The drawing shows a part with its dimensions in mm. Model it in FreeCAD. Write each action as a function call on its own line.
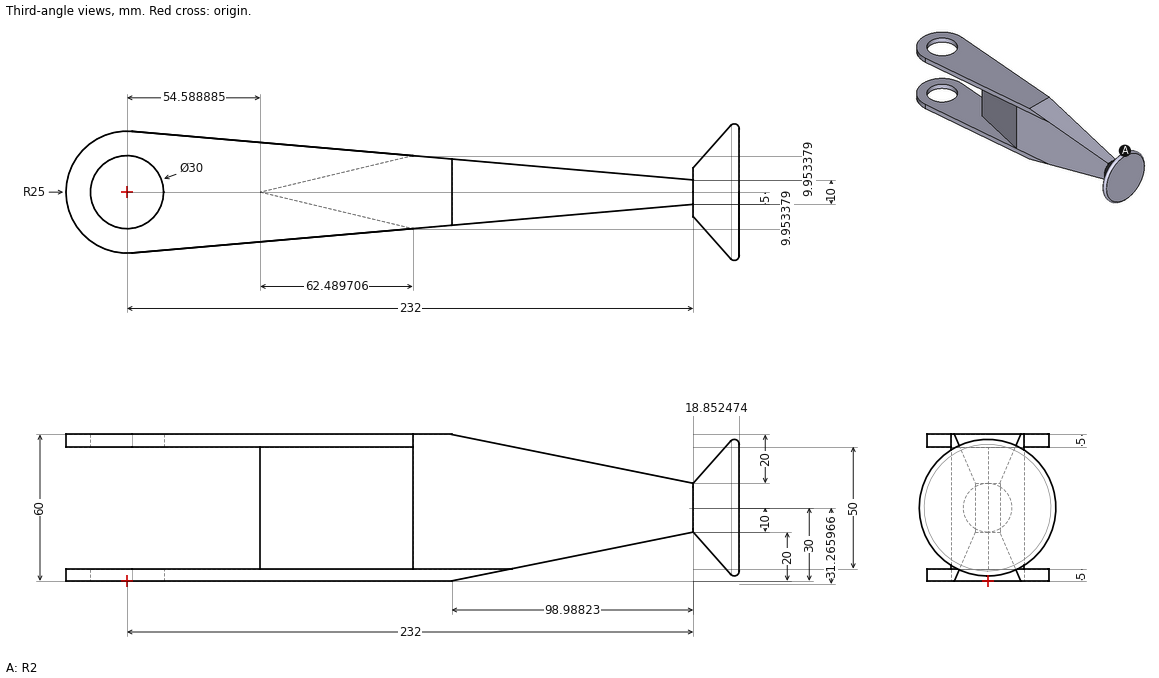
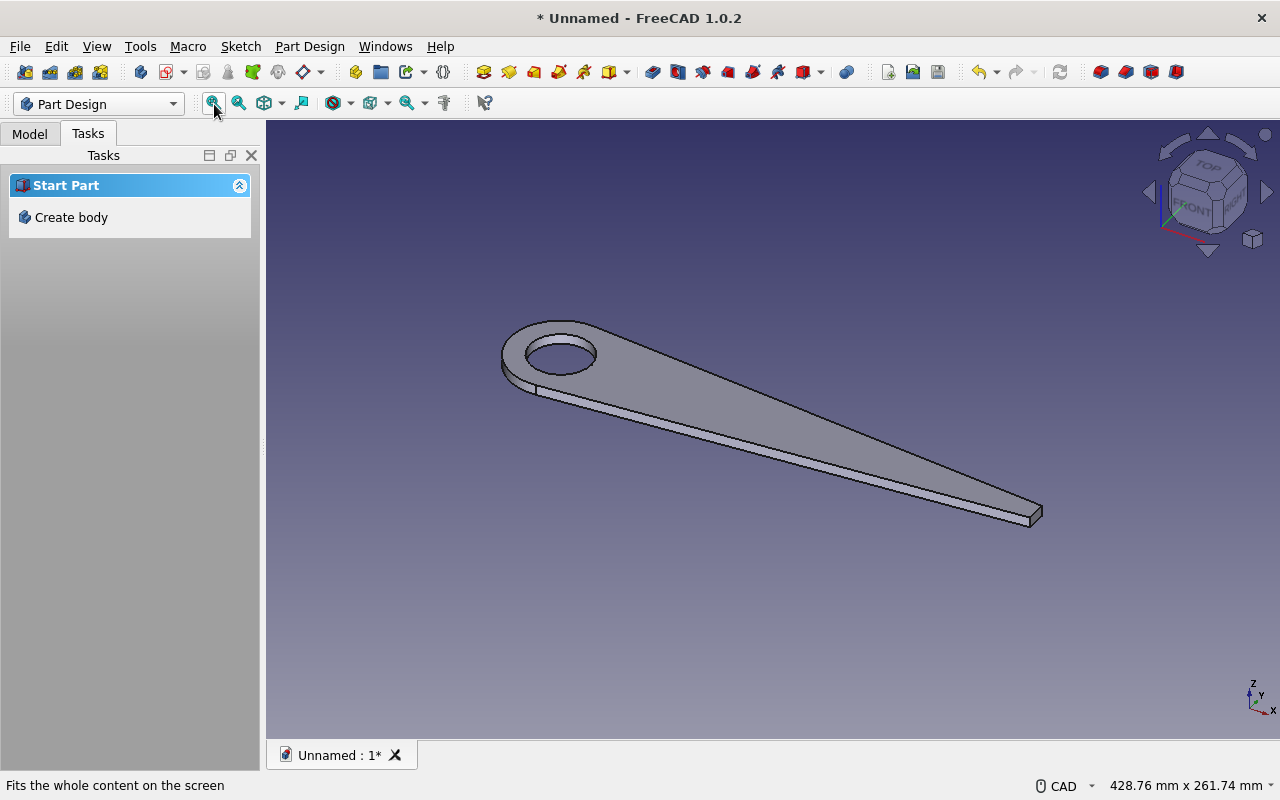
click(698, 399)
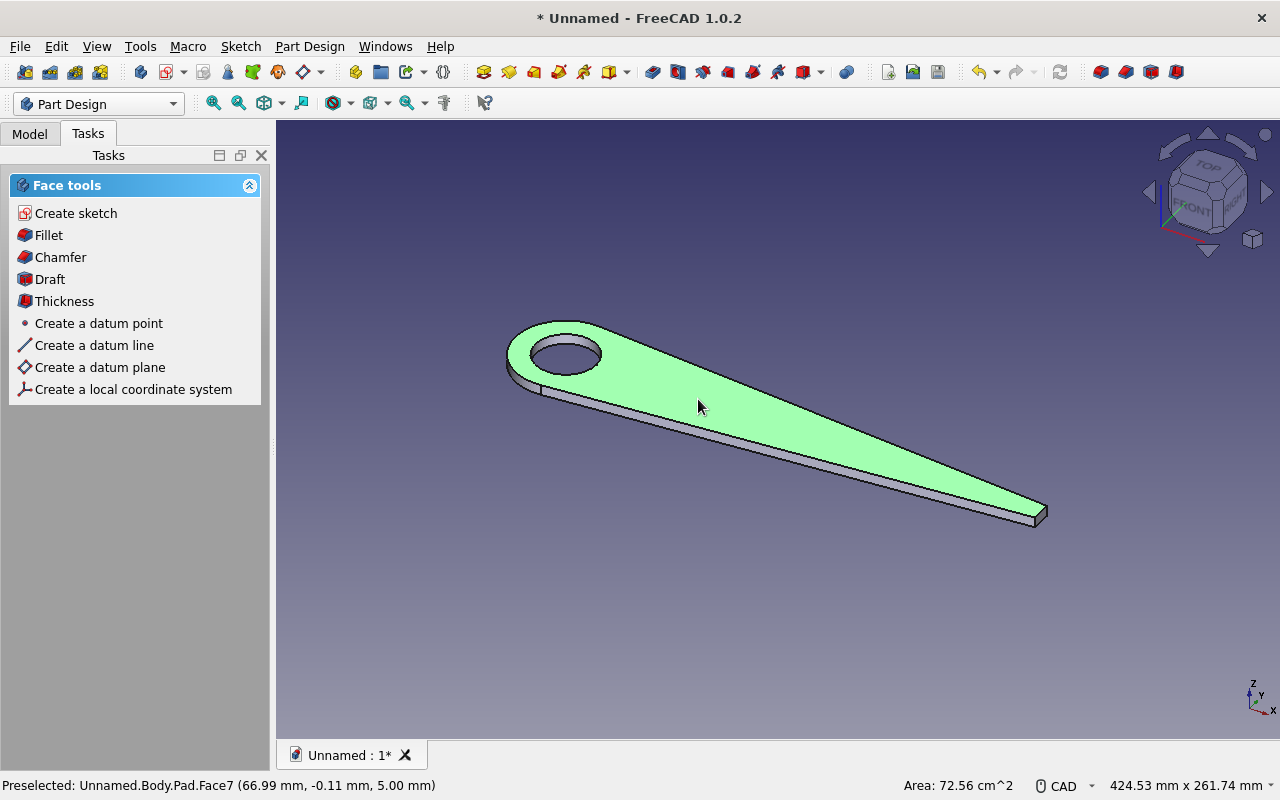
click(166, 72)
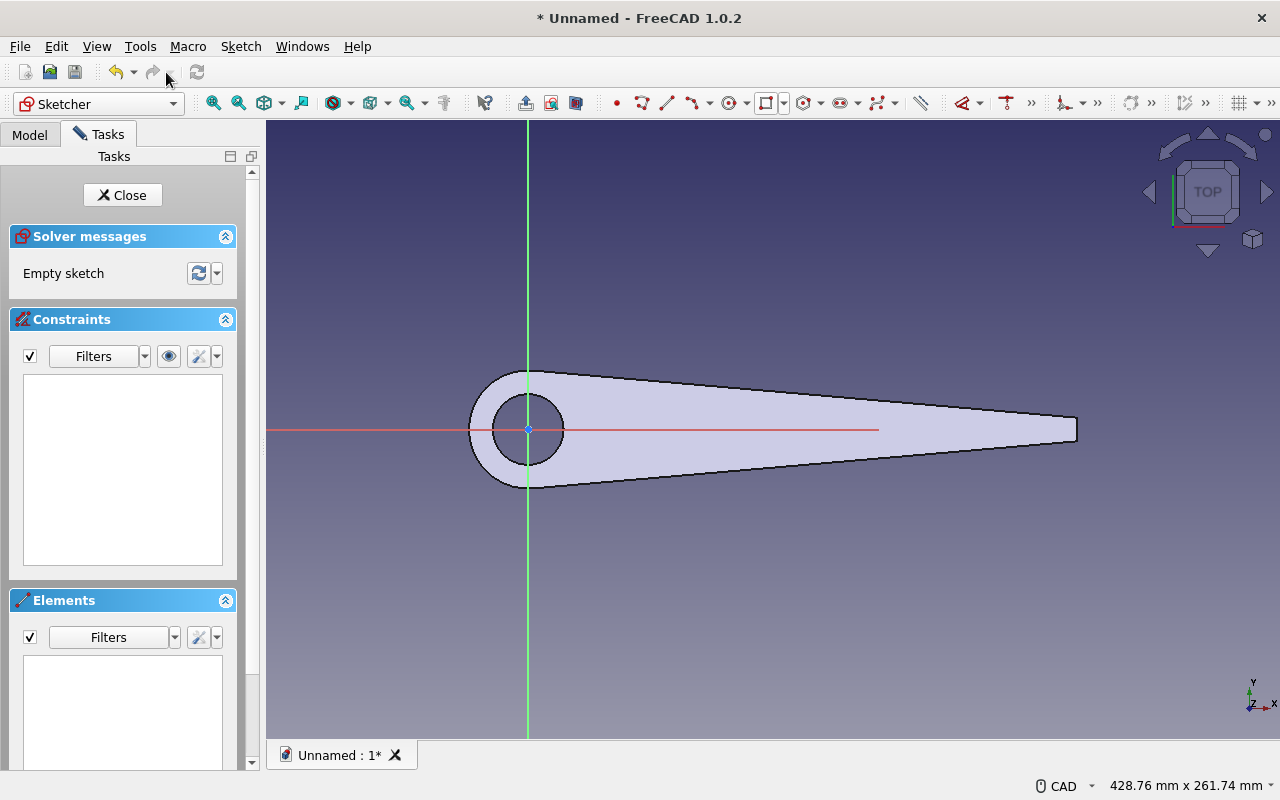
click(642, 104)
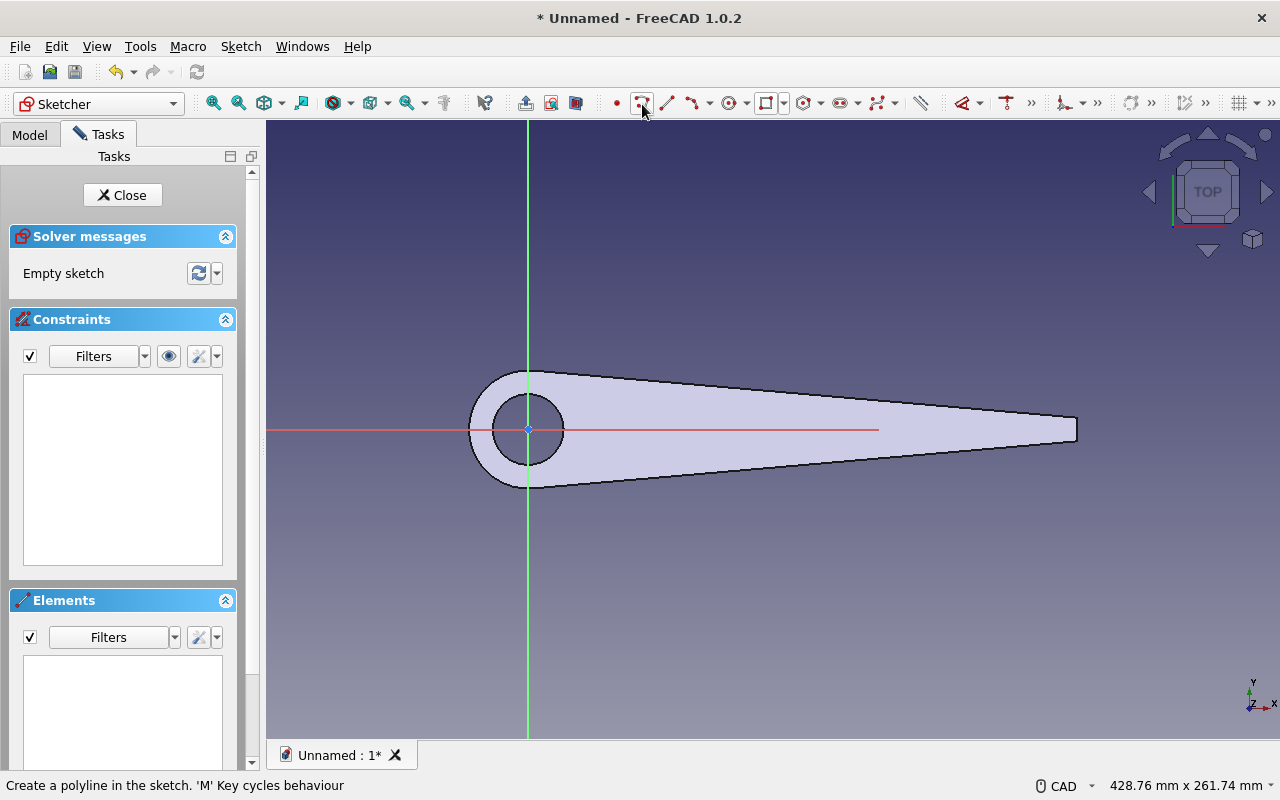
click(657, 430)
click(805, 465)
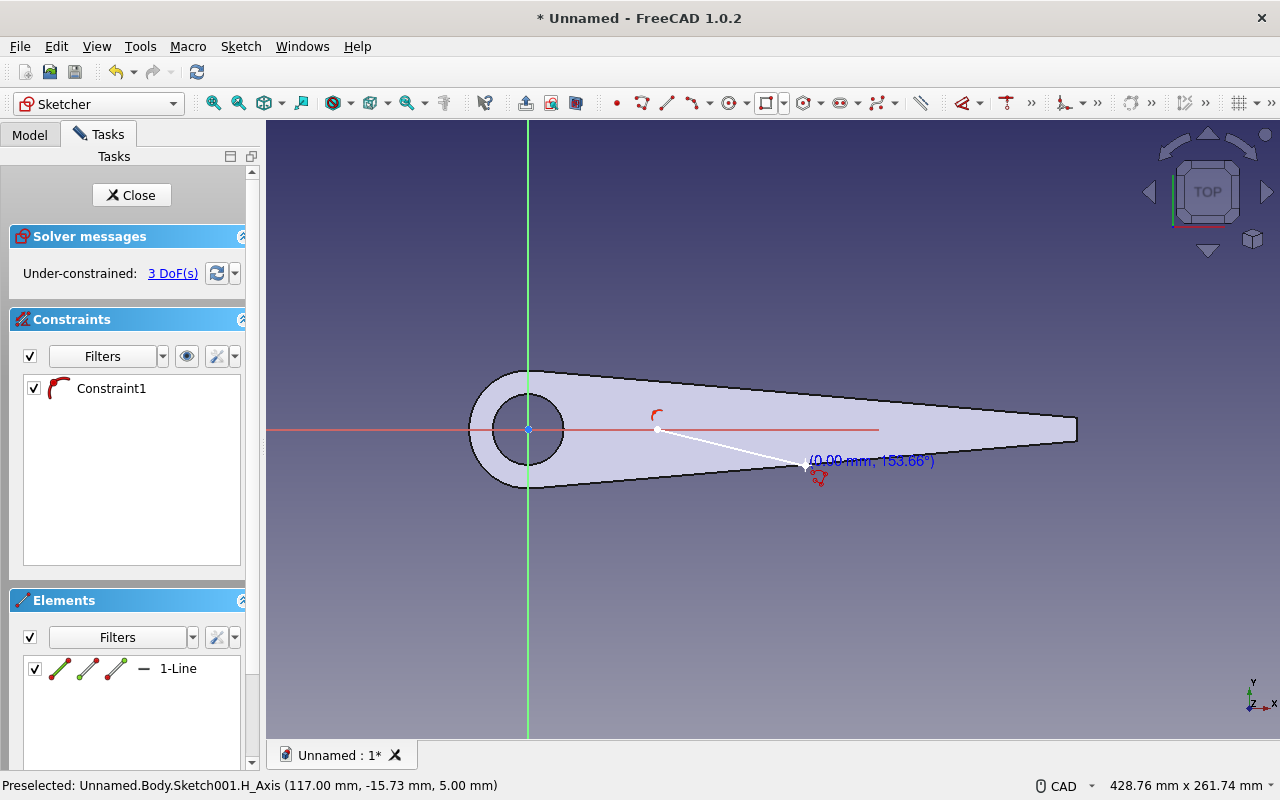
scroll(1077, 441, up, 2)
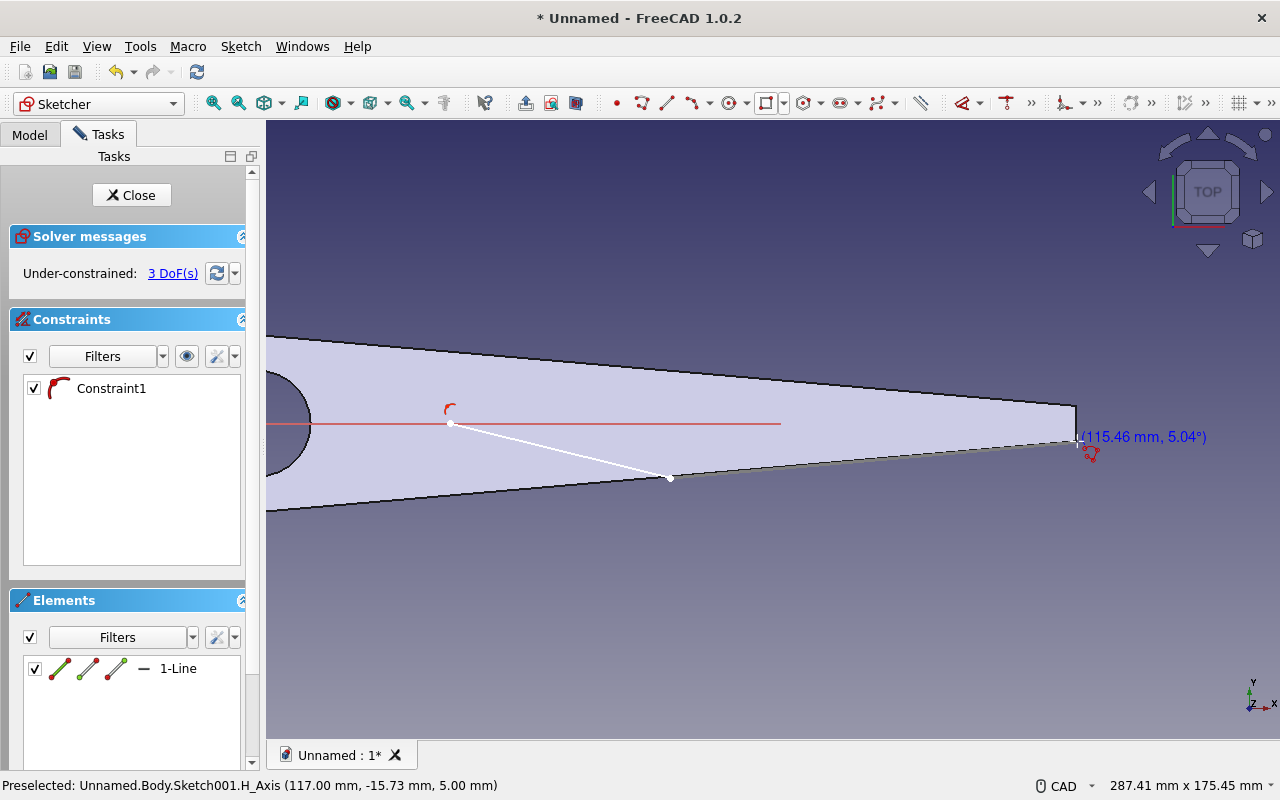
click(1076, 441)
click(1076, 406)
click(671, 371)
click(450, 424)
key(Escape)
key(Escape)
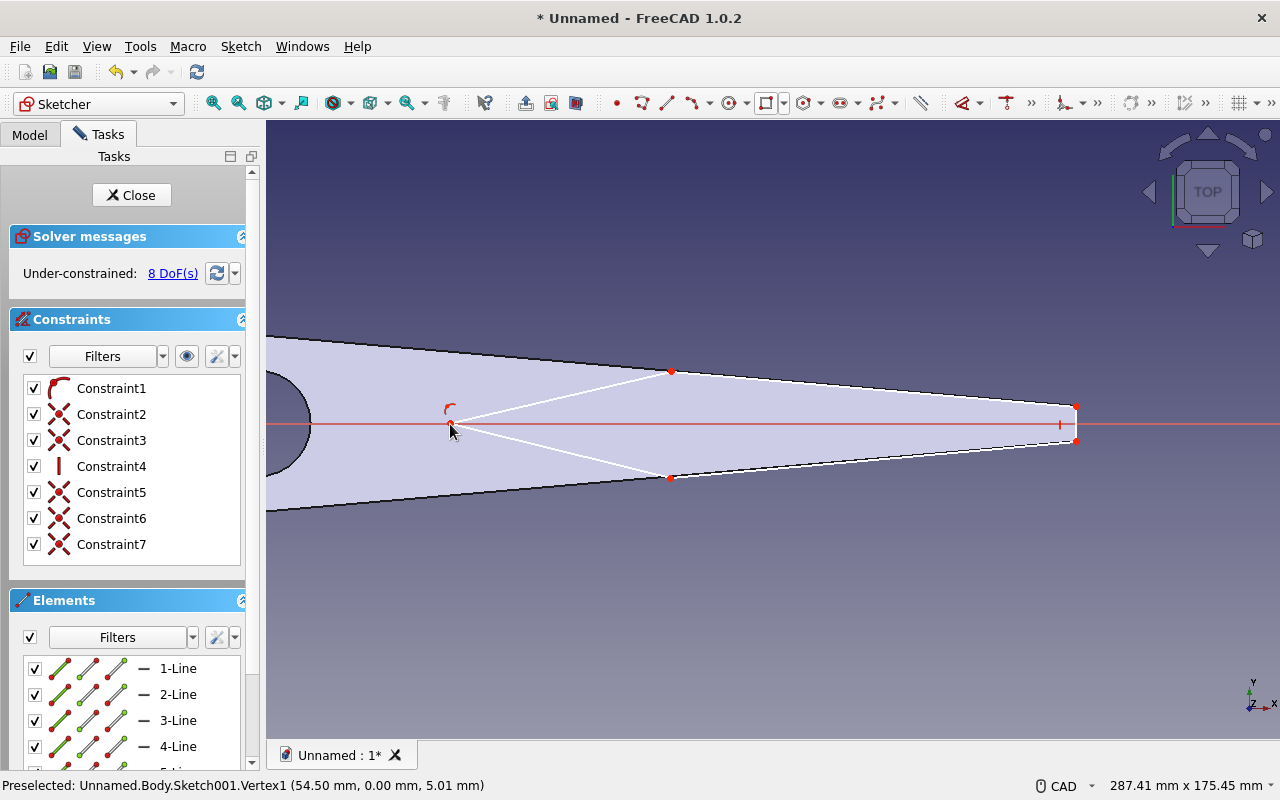
click(962, 104)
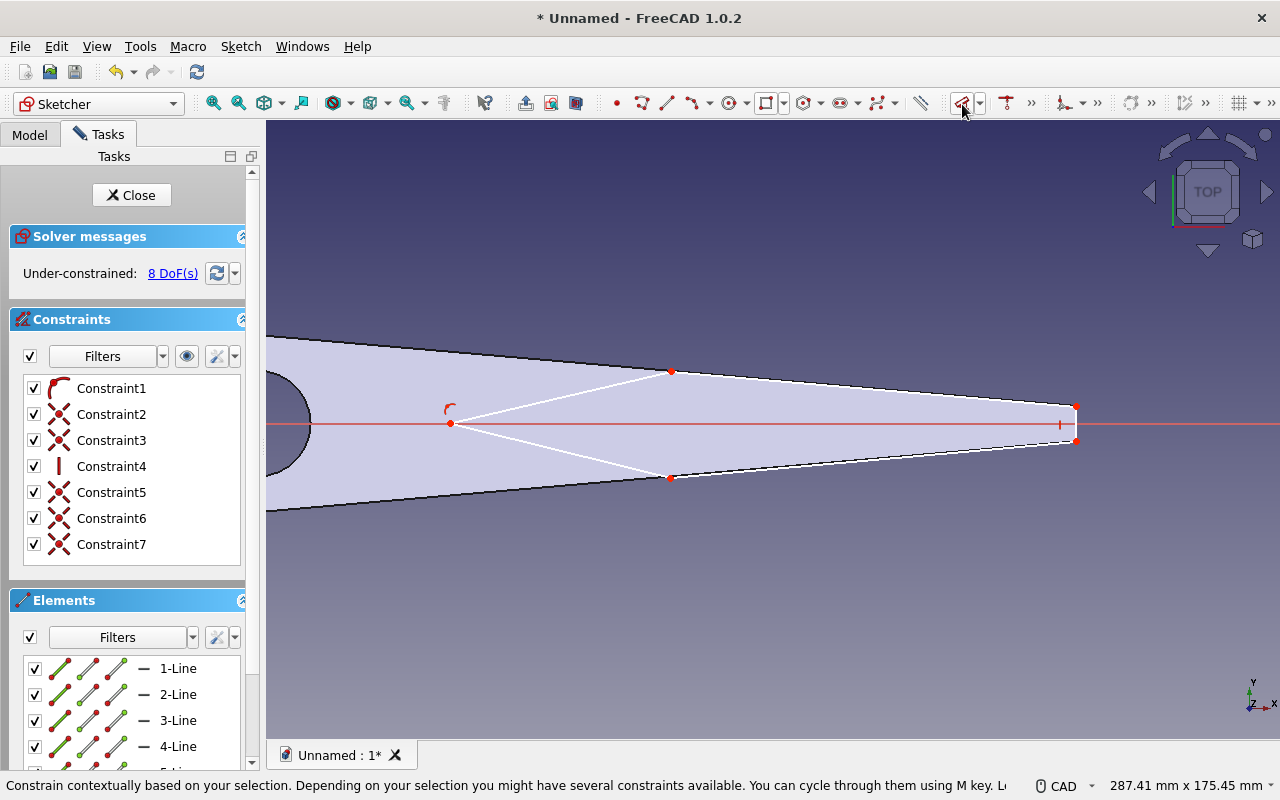
click(1076, 421)
click(1110, 437)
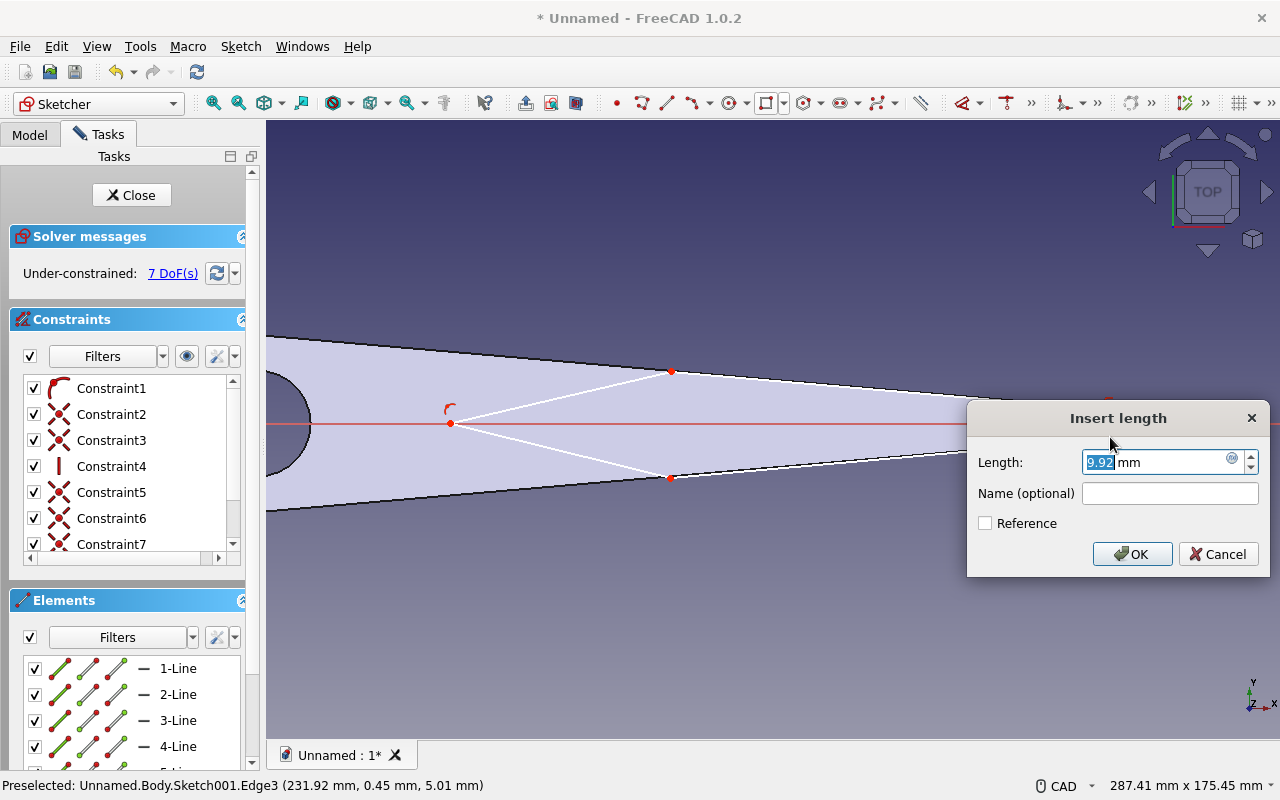
text(10)
key(Return)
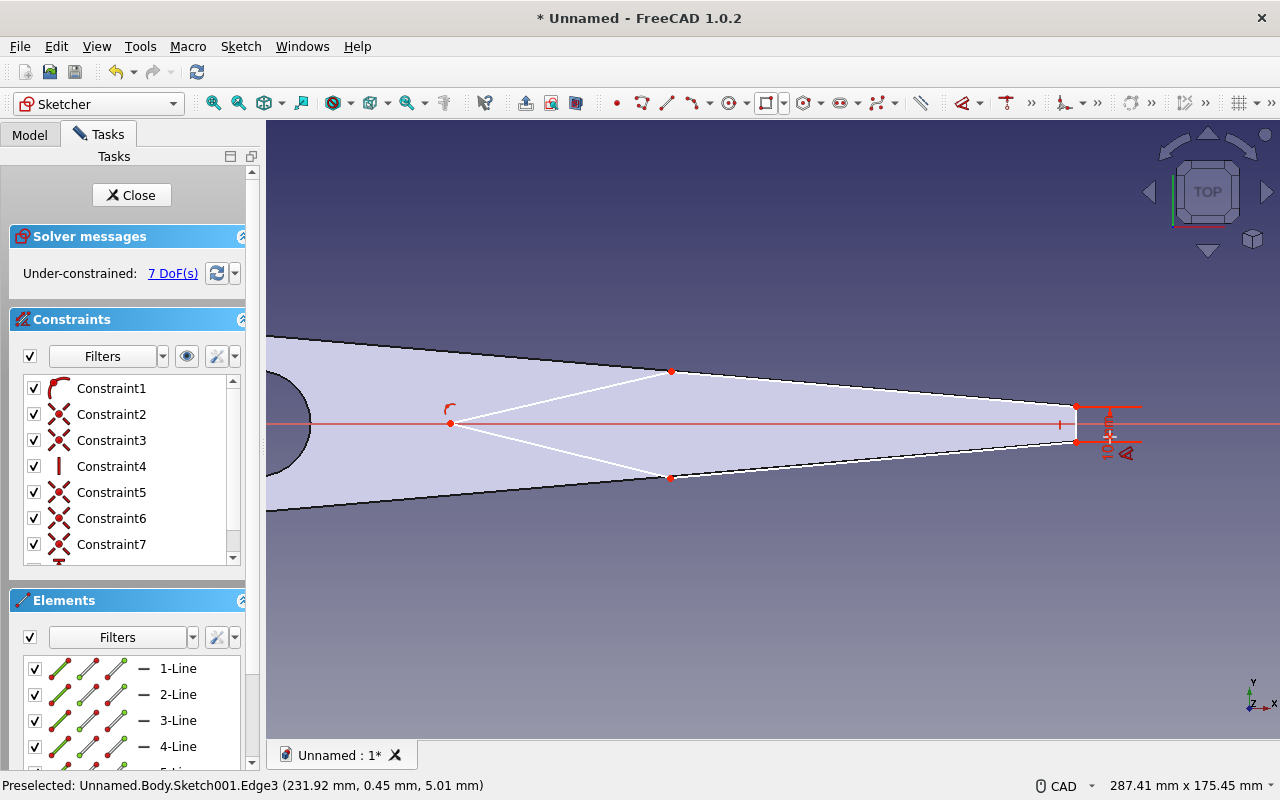
scroll(1076, 442, up, 5)